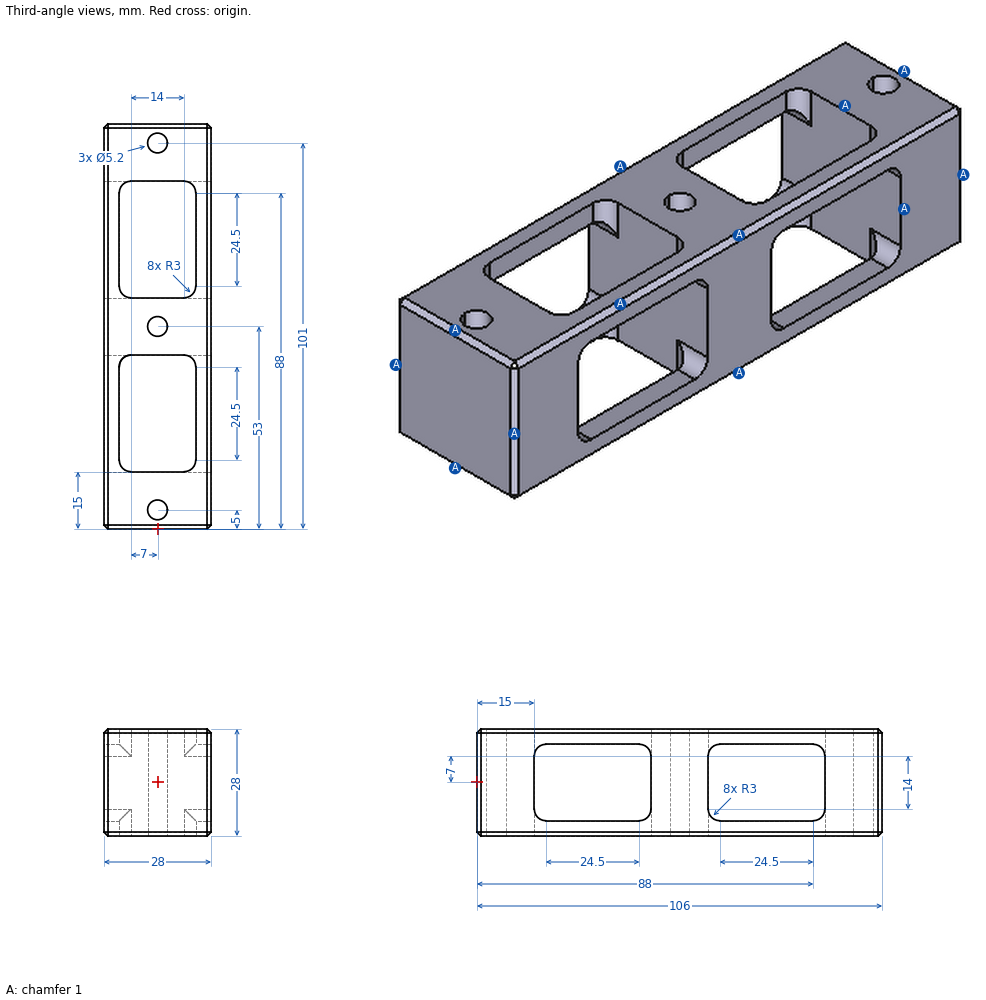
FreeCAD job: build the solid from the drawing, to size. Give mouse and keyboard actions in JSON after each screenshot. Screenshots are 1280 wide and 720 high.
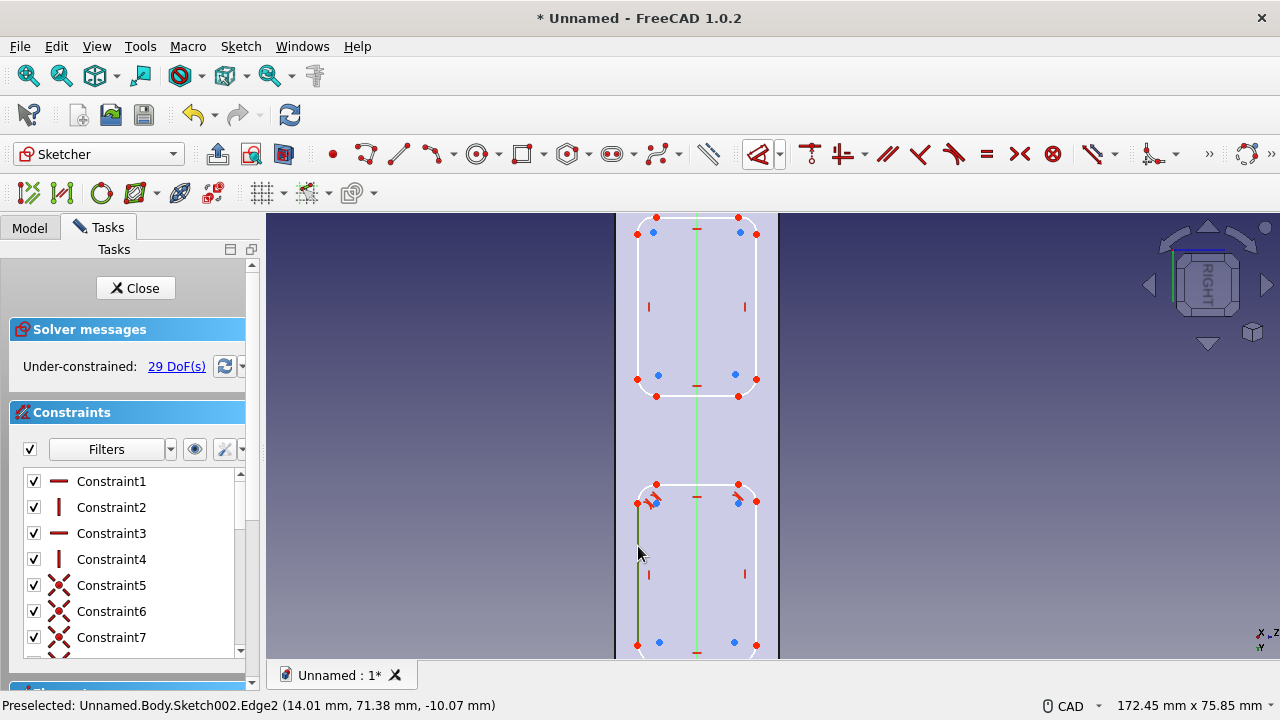
{"action": "scroll", "coordinate": [713, 486], "scroll_direction": "down", "scroll_amount": 3}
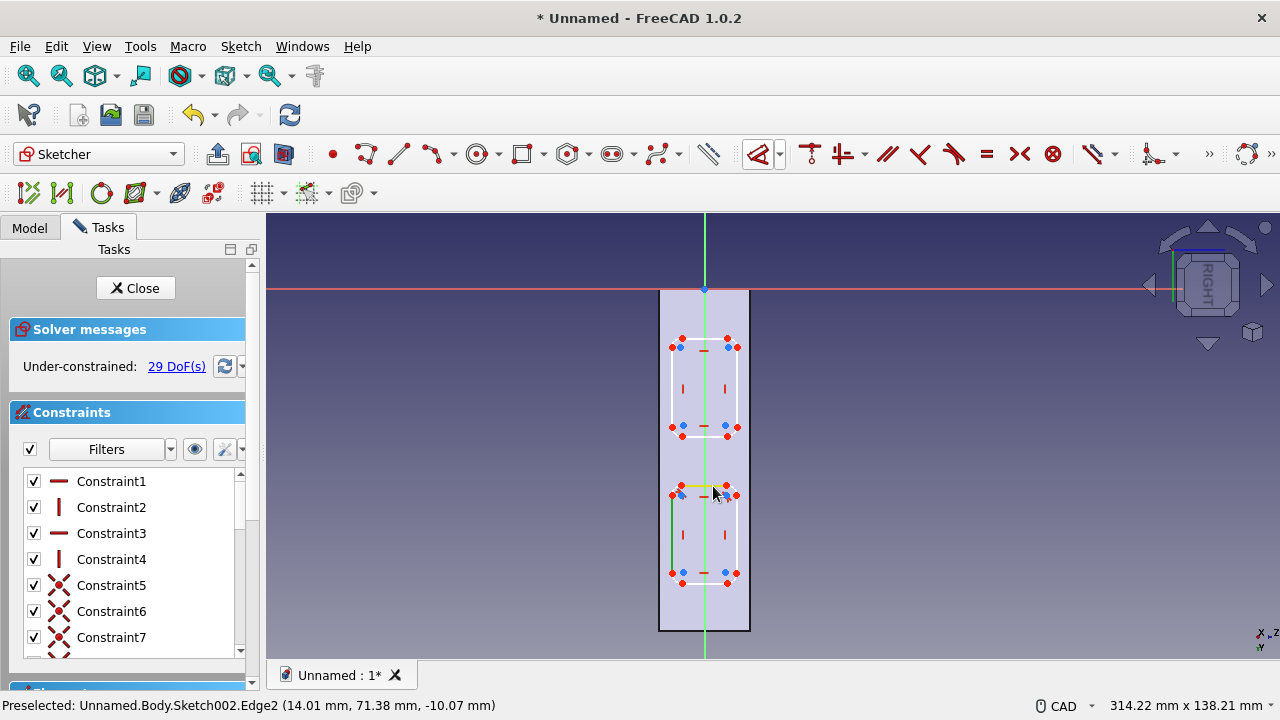
{"action": "scroll", "coordinate": [675, 581], "scroll_direction": "up", "scroll_amount": 4}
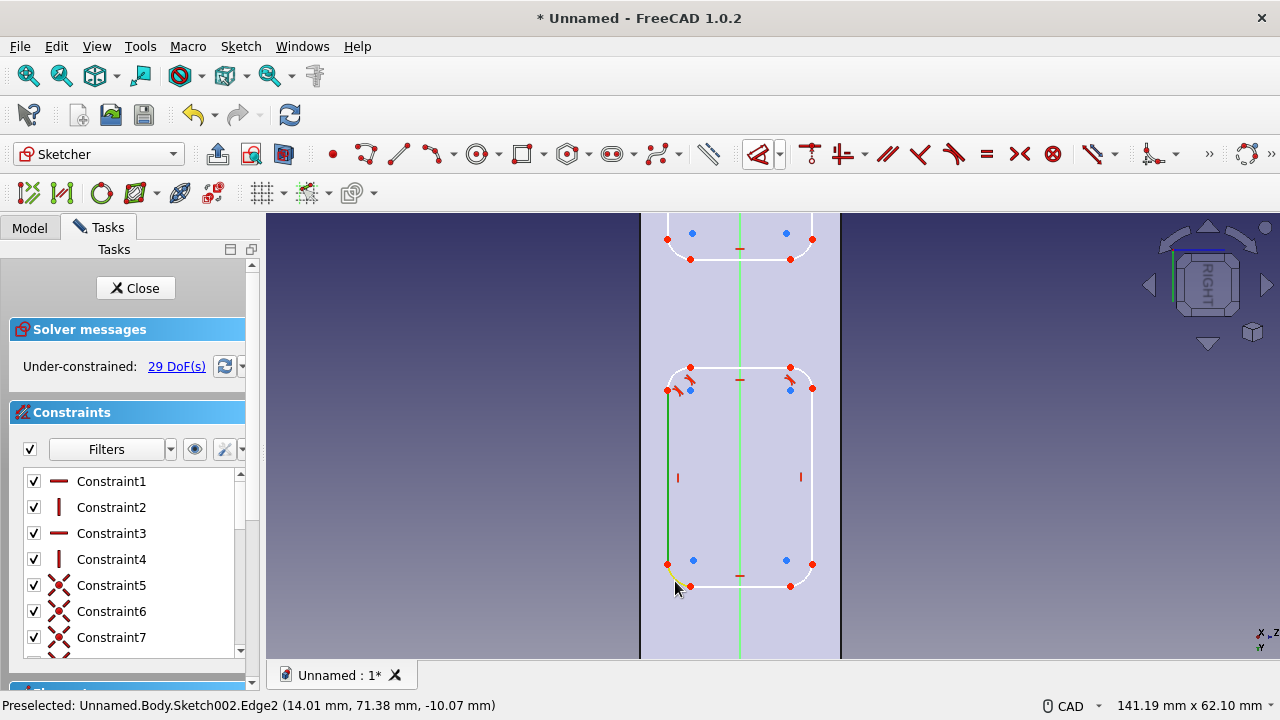
{"action": "left_click", "coordinate": [675, 579]}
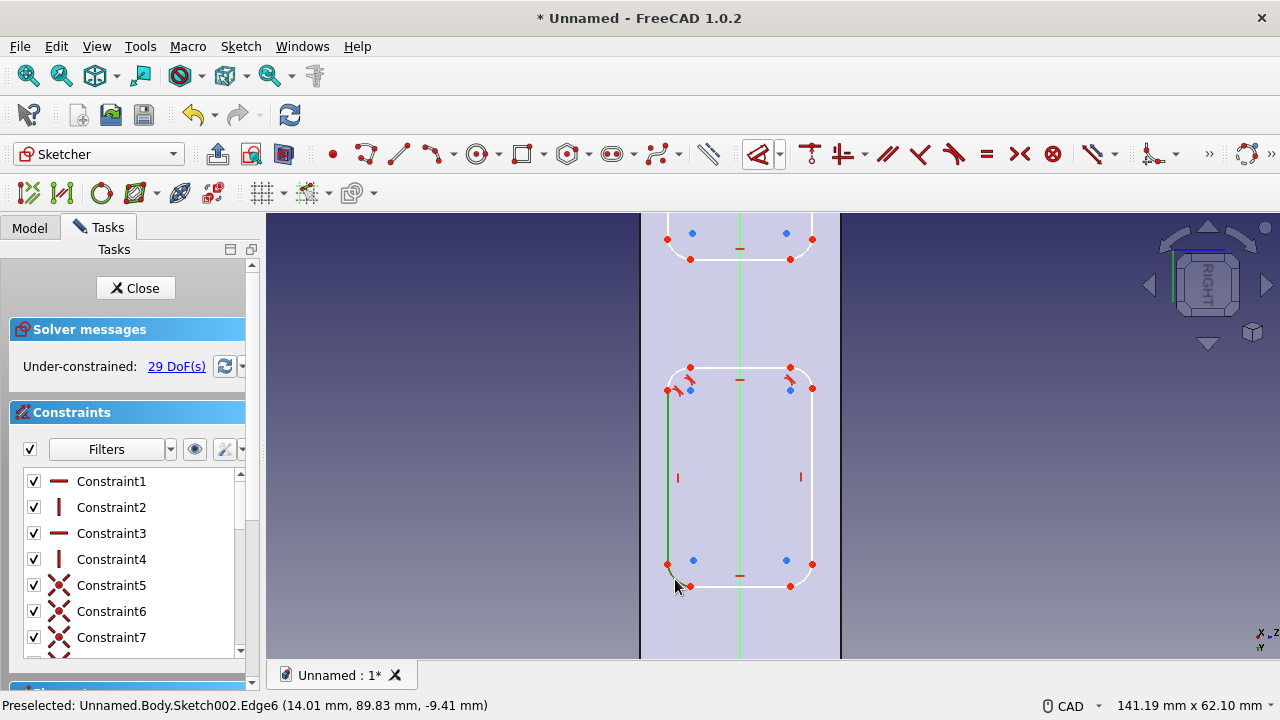
{"action": "key", "text": "t"}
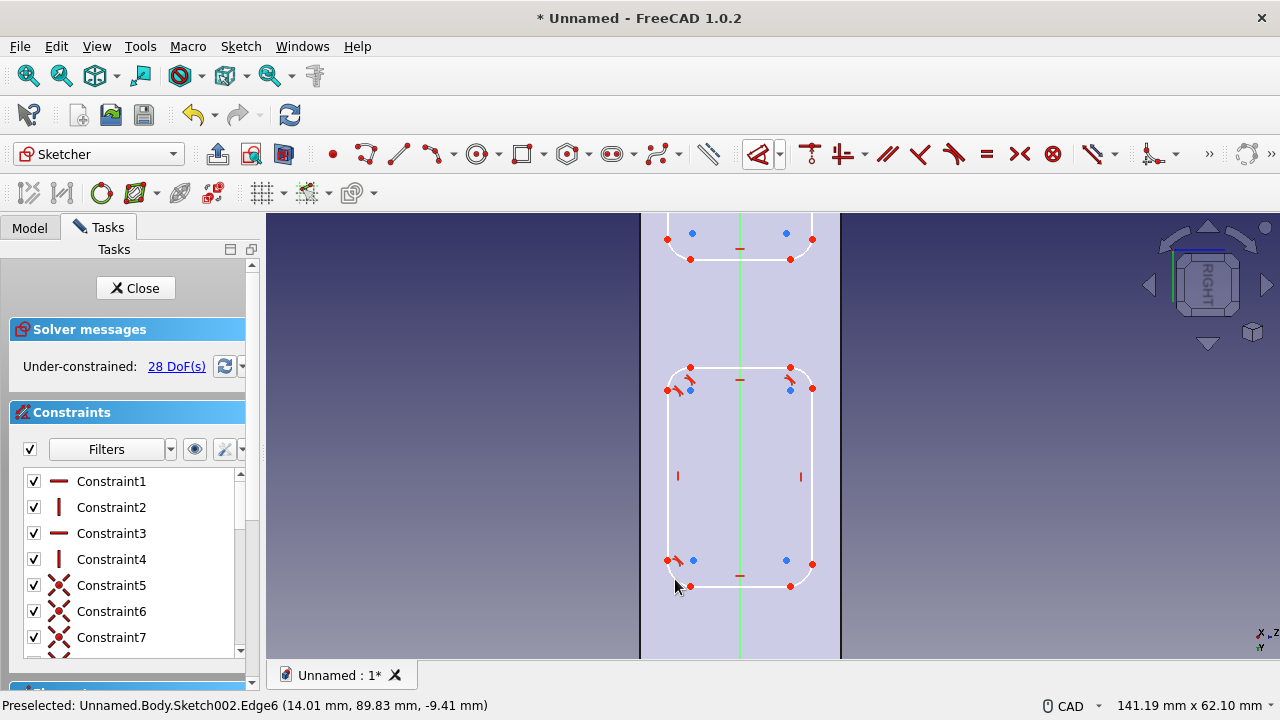
{"action": "left_click", "coordinate": [720, 587]}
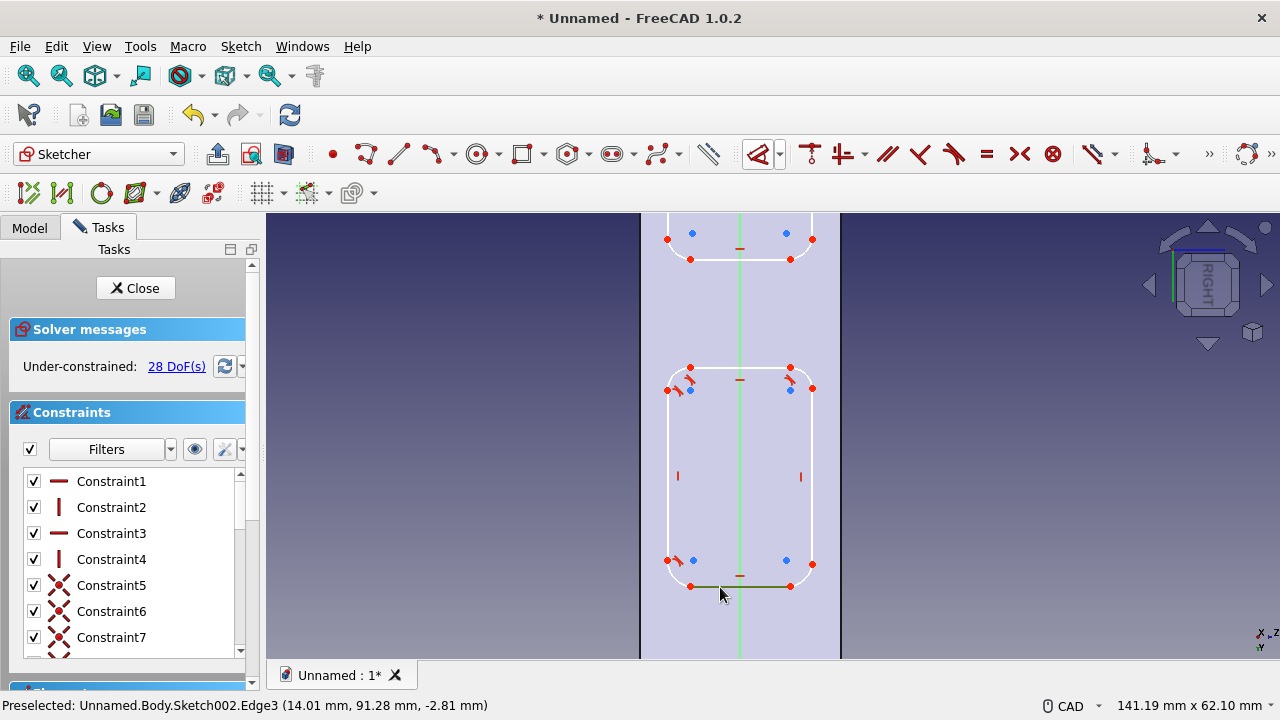
{"action": "scroll", "coordinate": [670, 572], "scroll_direction": "up", "scroll_amount": 2}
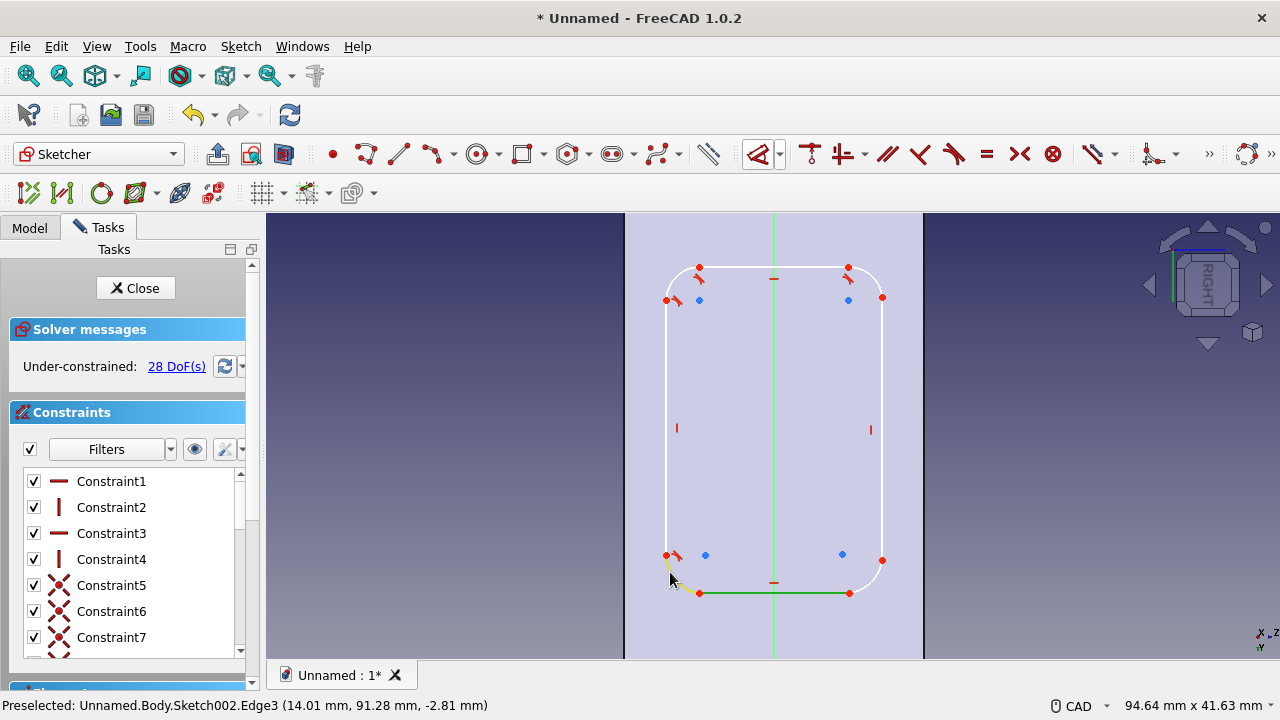
{"action": "left_click", "coordinate": [670, 571]}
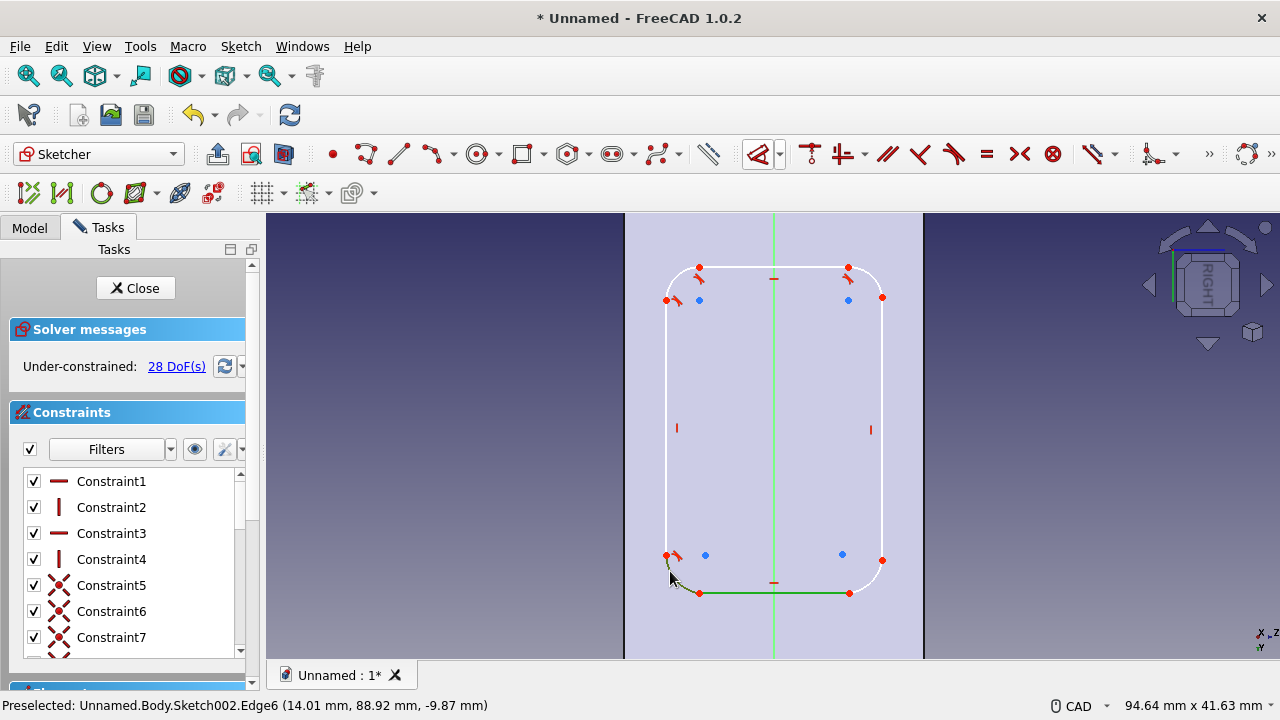
{"action": "left_click", "coordinate": [954, 154]}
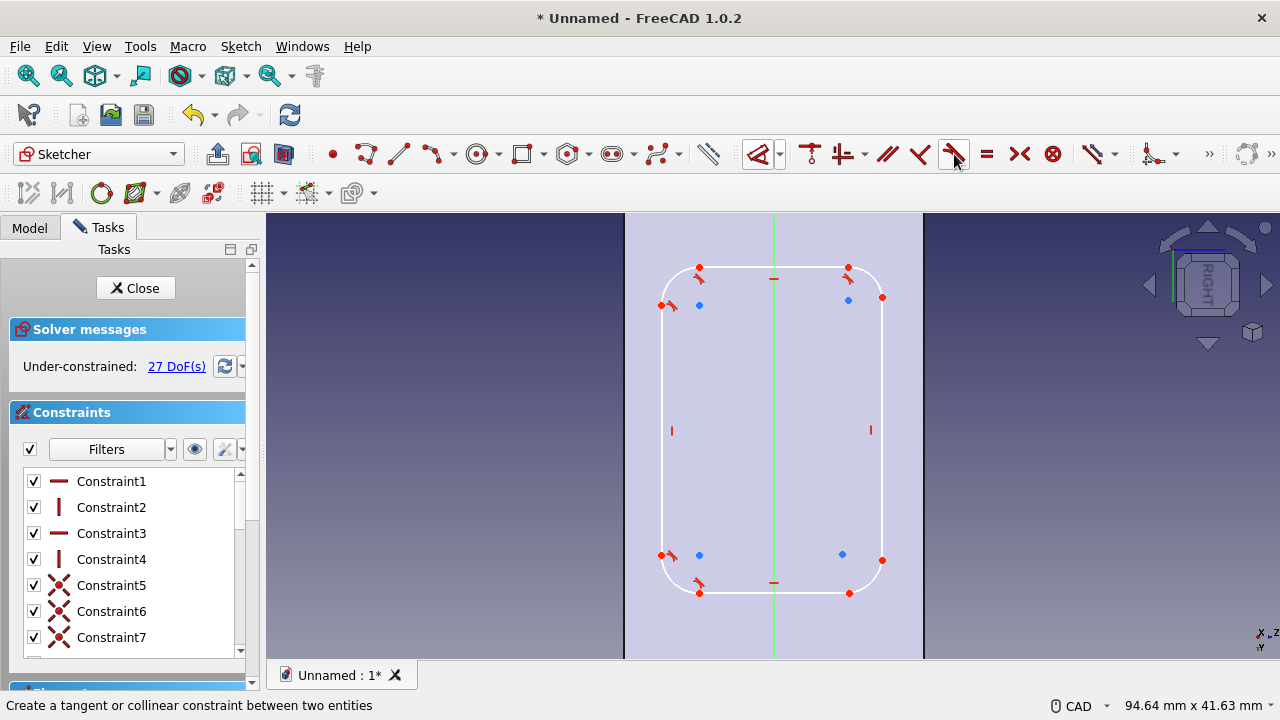
{"action": "left_click", "coordinate": [745, 593]}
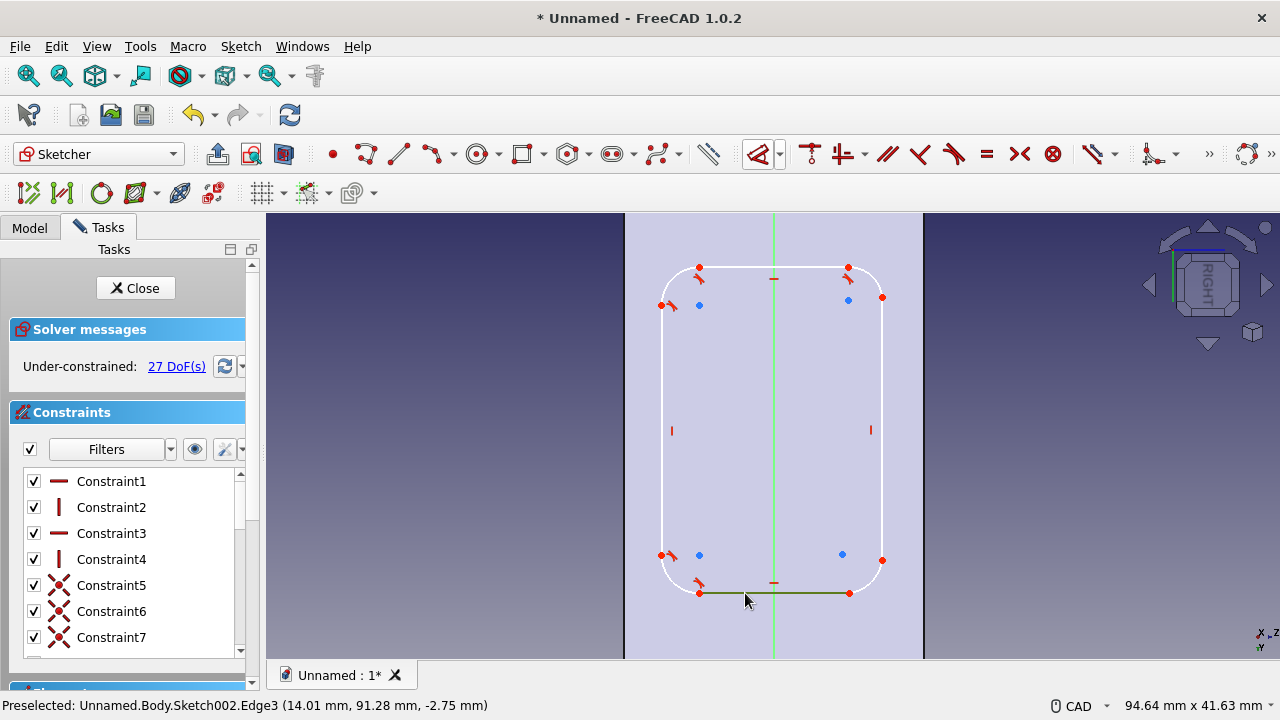
{"action": "left_click", "coordinate": [863, 588]}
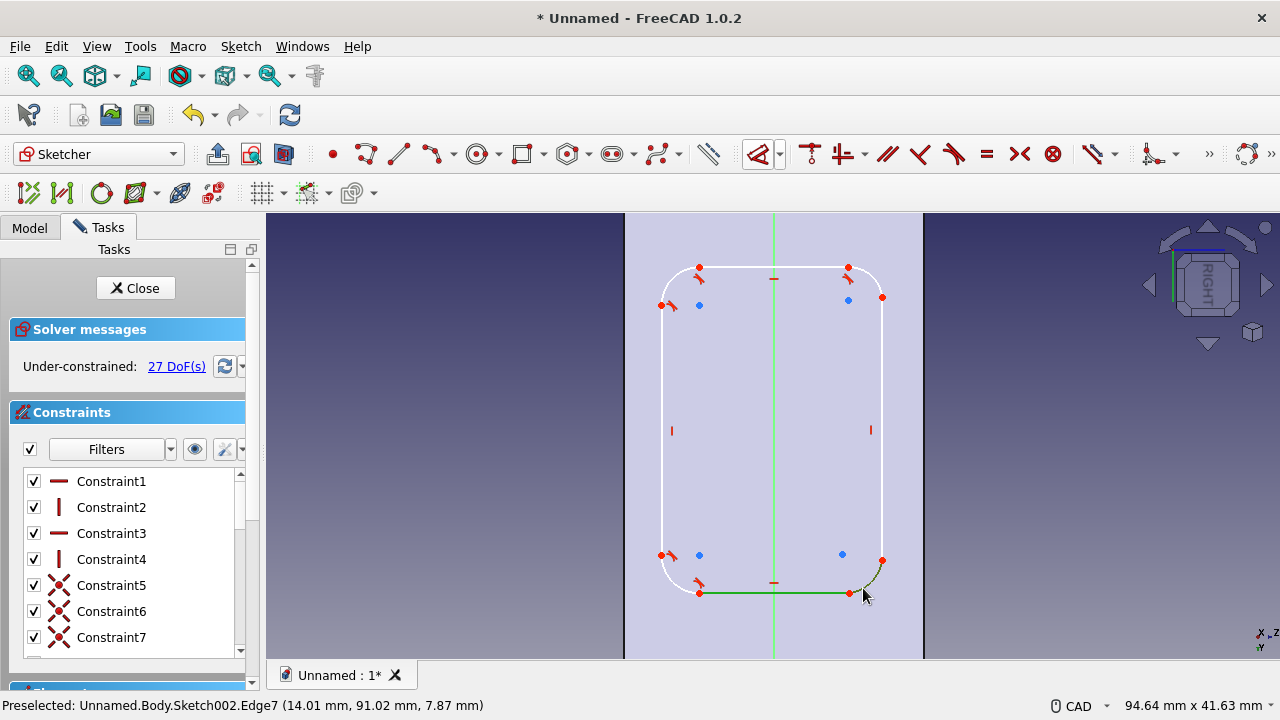
{"action": "left_click", "coordinate": [954, 154]}